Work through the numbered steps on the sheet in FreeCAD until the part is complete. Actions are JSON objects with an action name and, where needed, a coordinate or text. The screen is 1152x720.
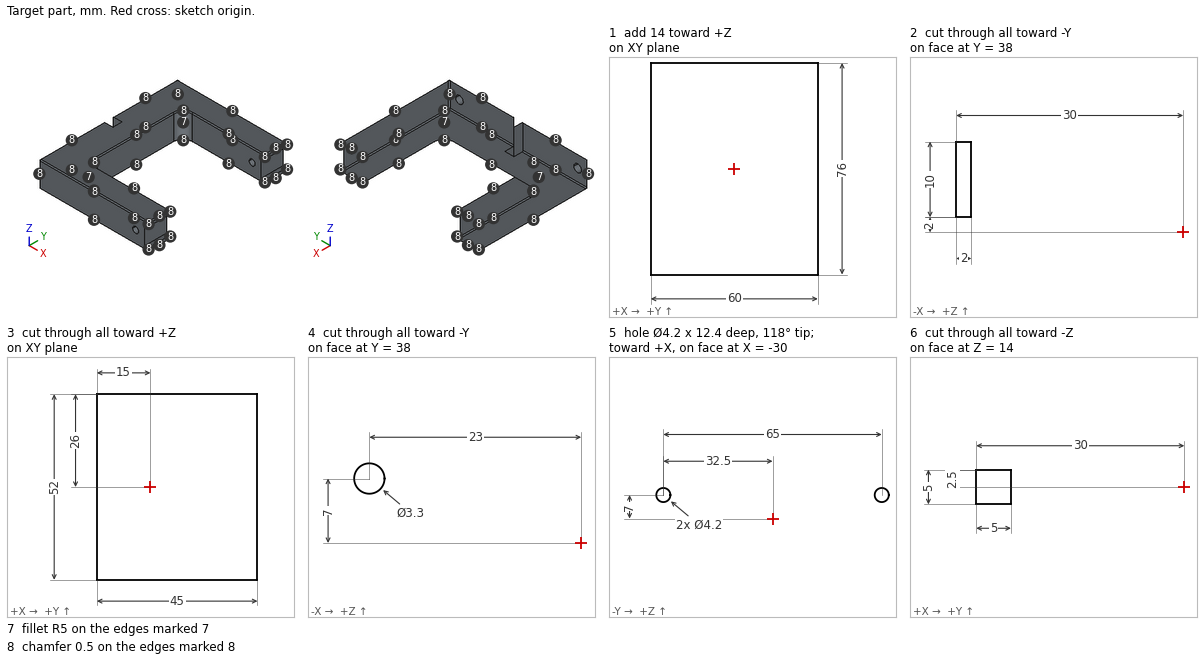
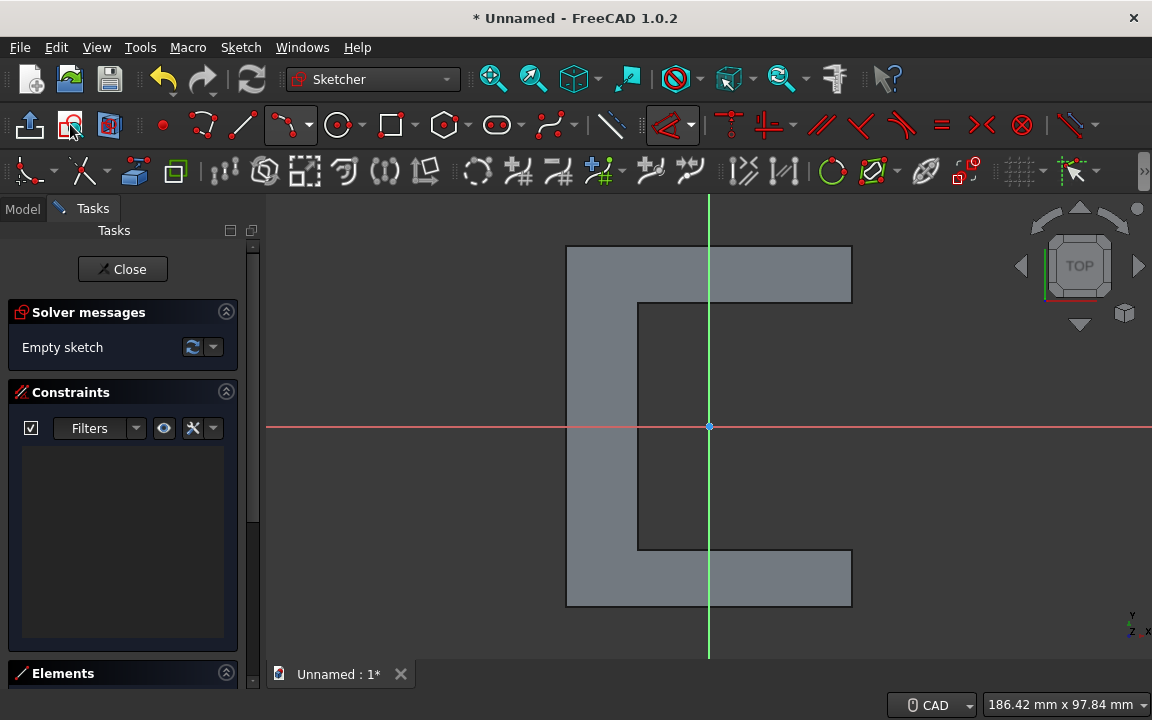
{"action": "scroll", "coordinate": [572, 427], "scroll_direction": "up", "scroll_amount": 12}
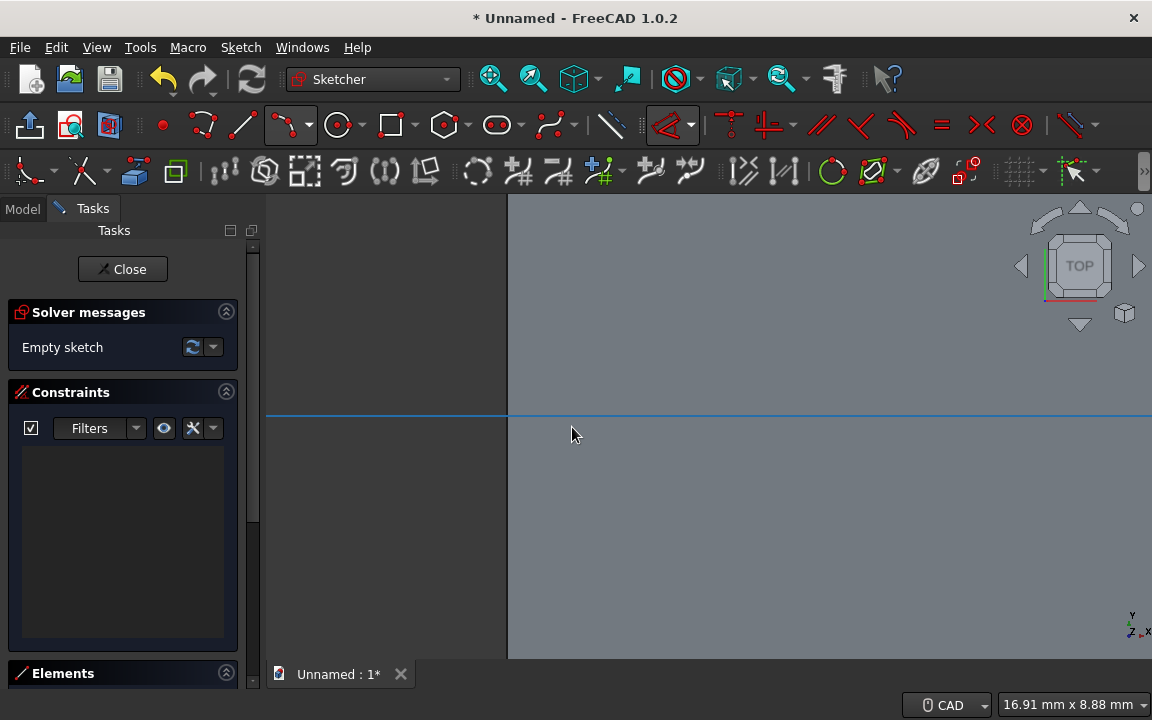
{"action": "key", "text": "g r"}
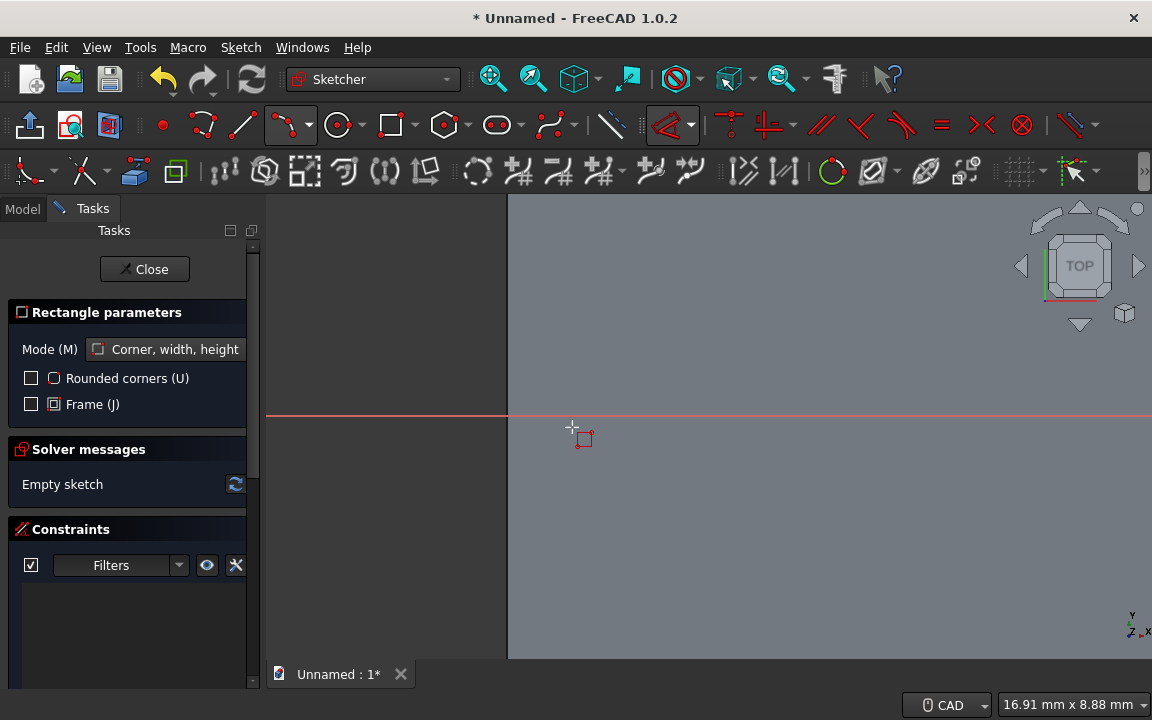
{"action": "left_click", "coordinate": [507, 285]}
{"action": "left_click", "coordinate": [769, 547]}
{"action": "key", "text": "Escape"}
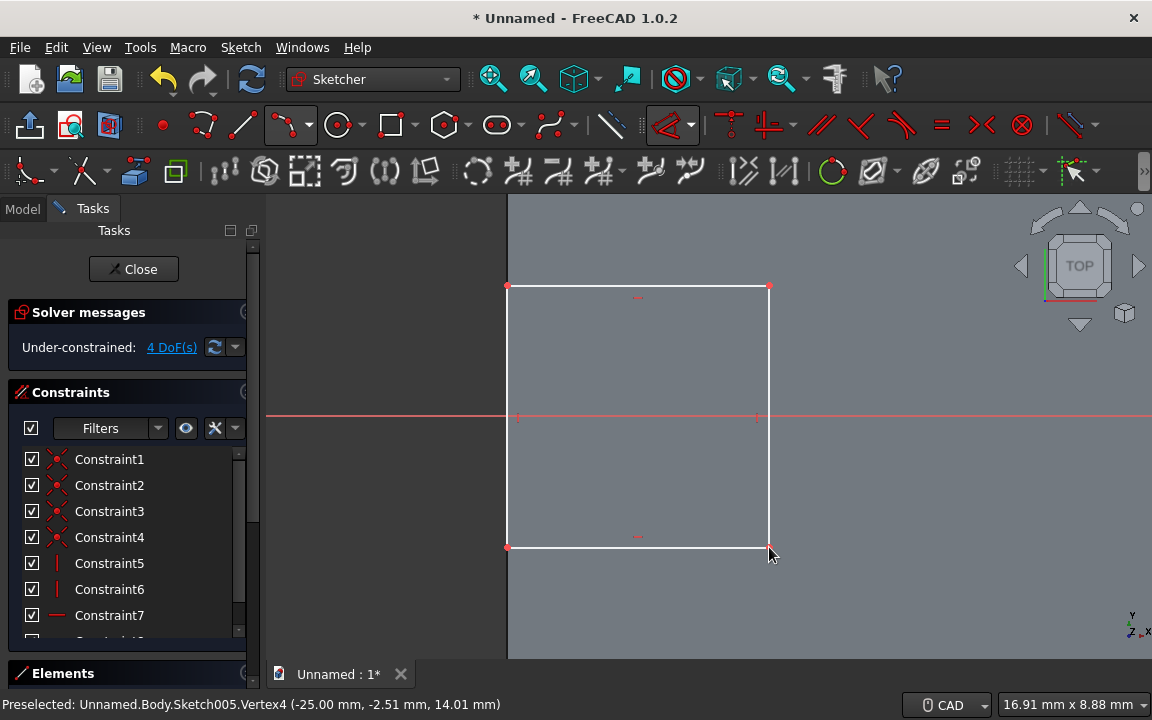
{"action": "left_click", "coordinate": [507, 365]}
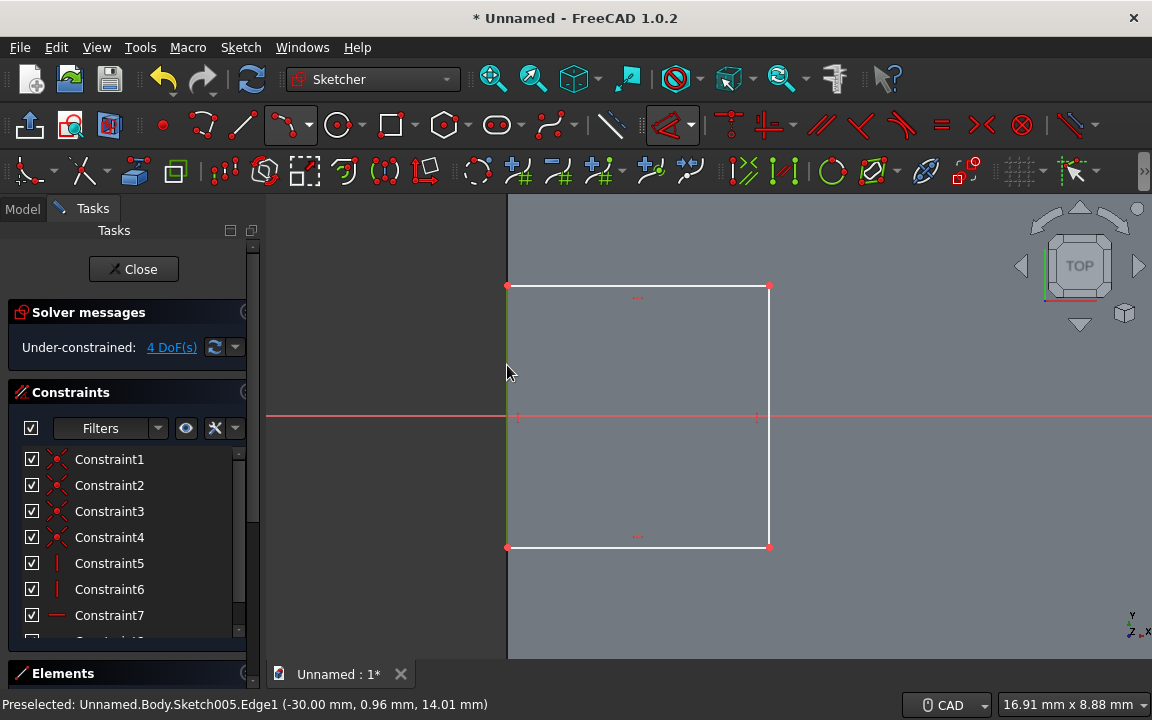
{"action": "key", "text": "i"}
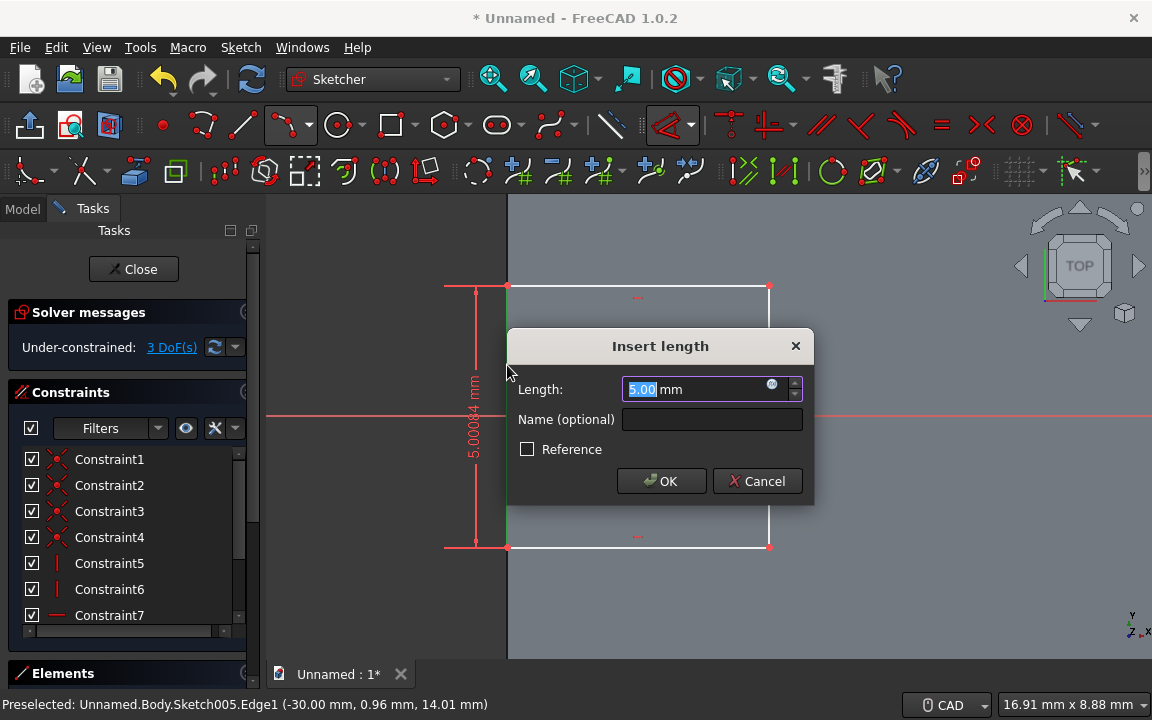
{"action": "type", "text": "5"}
{"action": "key", "text": "Return"}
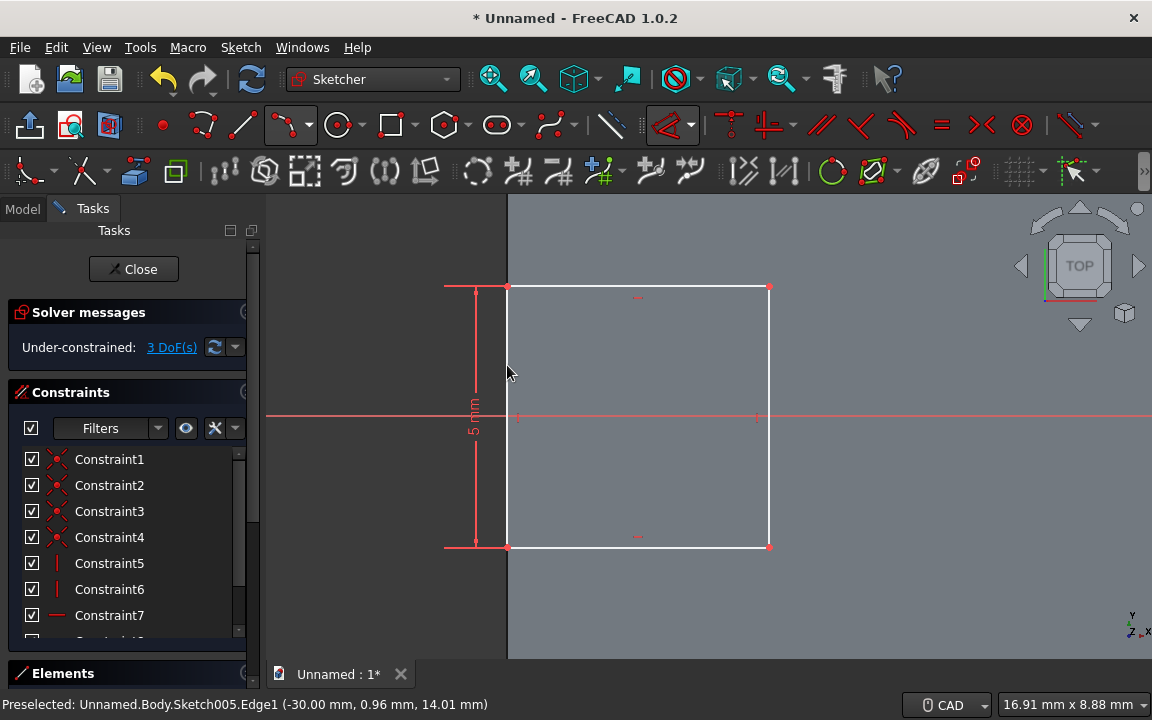
{"action": "left_click", "coordinate": [586, 548]}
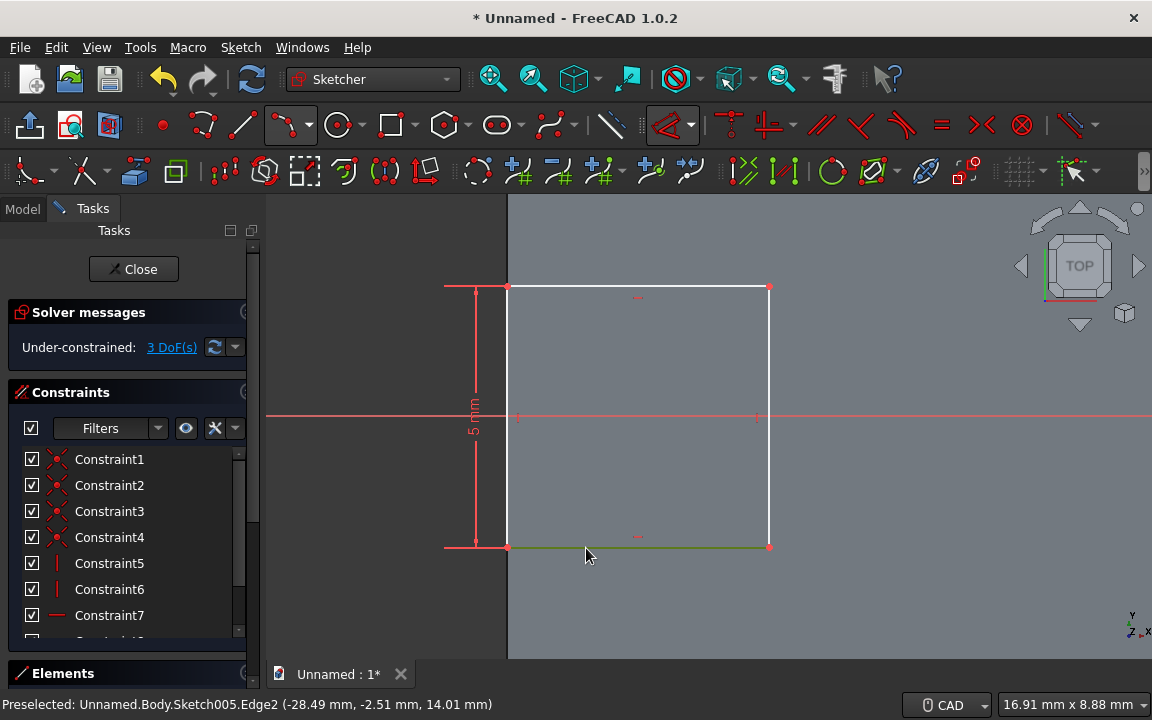
{"action": "left_click", "coordinate": [694, 126]}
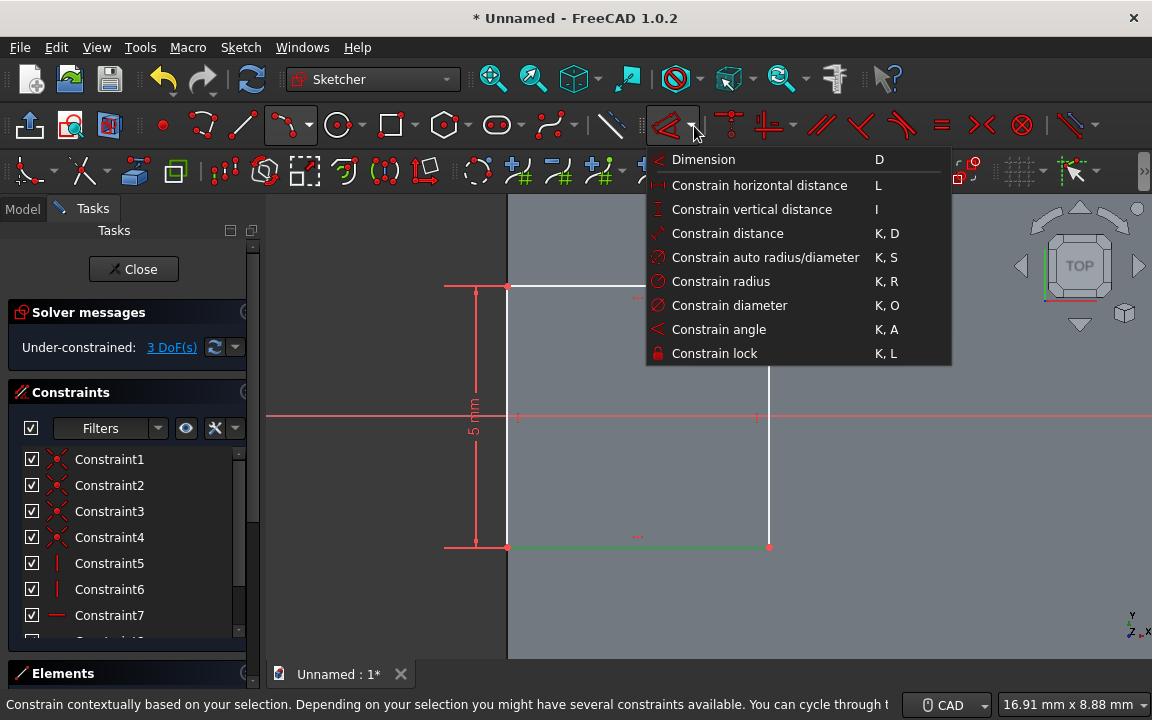
{"action": "left_click", "coordinate": [799, 185]}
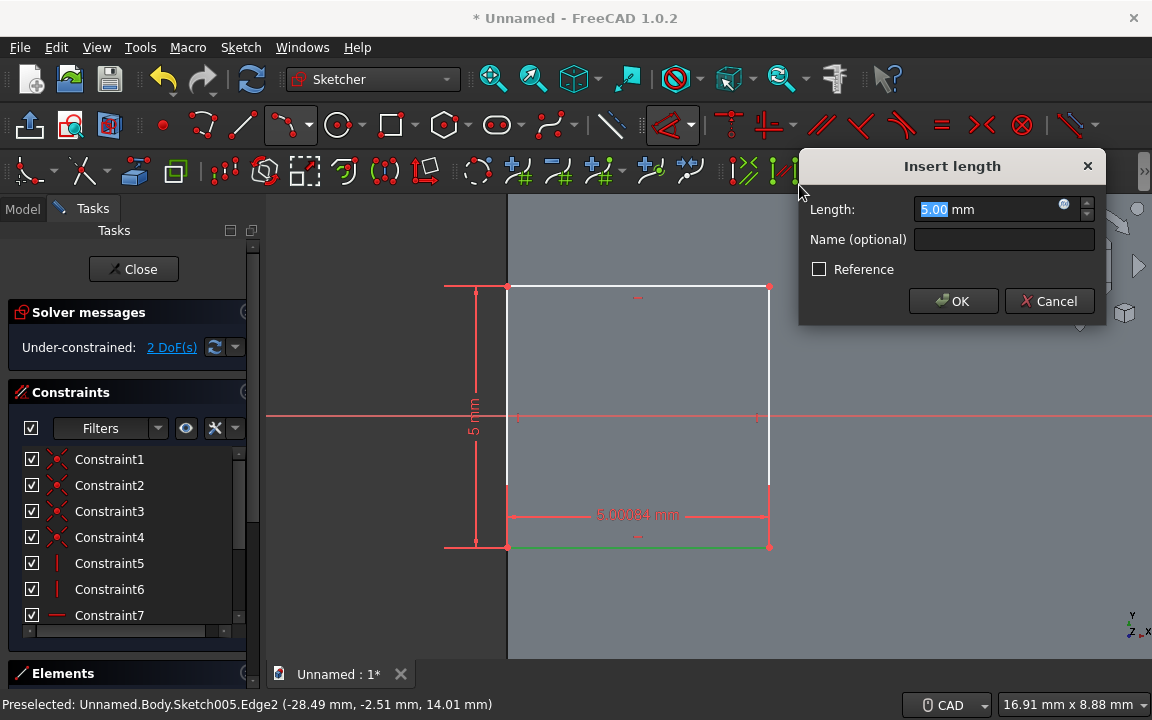
{"action": "type", "text": "5"}
{"action": "key", "text": "Return"}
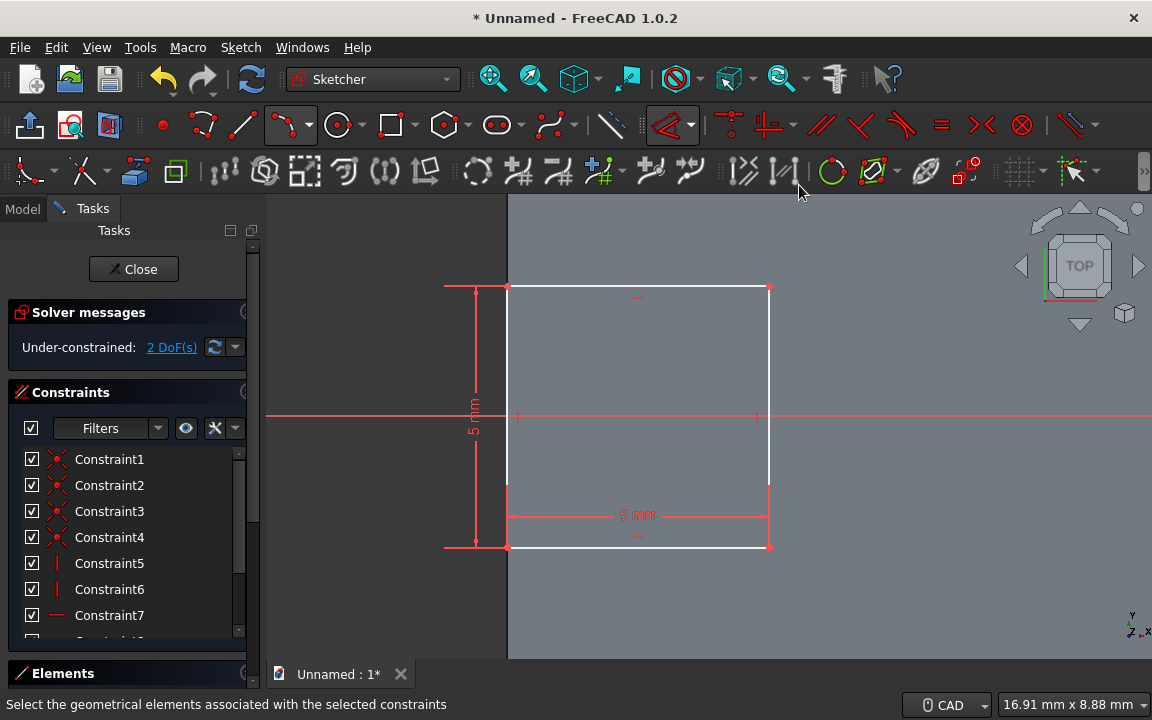
{"action": "left_click", "coordinate": [507, 286]}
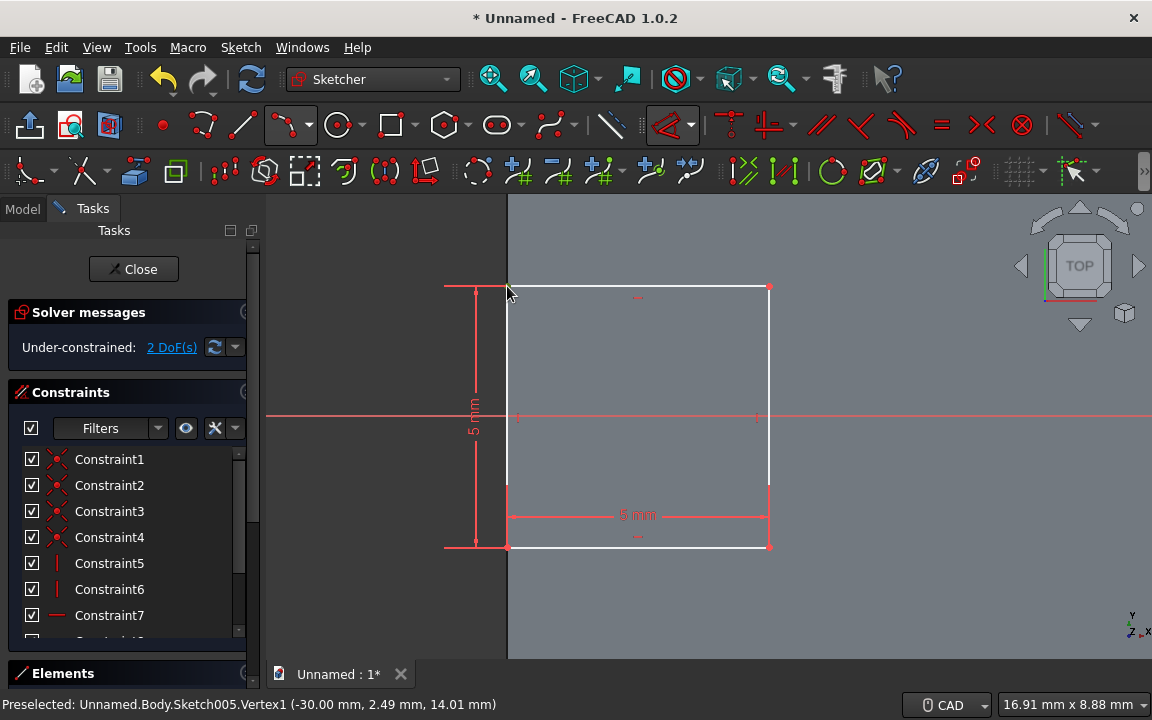
{"action": "left_click", "coordinate": [694, 126]}